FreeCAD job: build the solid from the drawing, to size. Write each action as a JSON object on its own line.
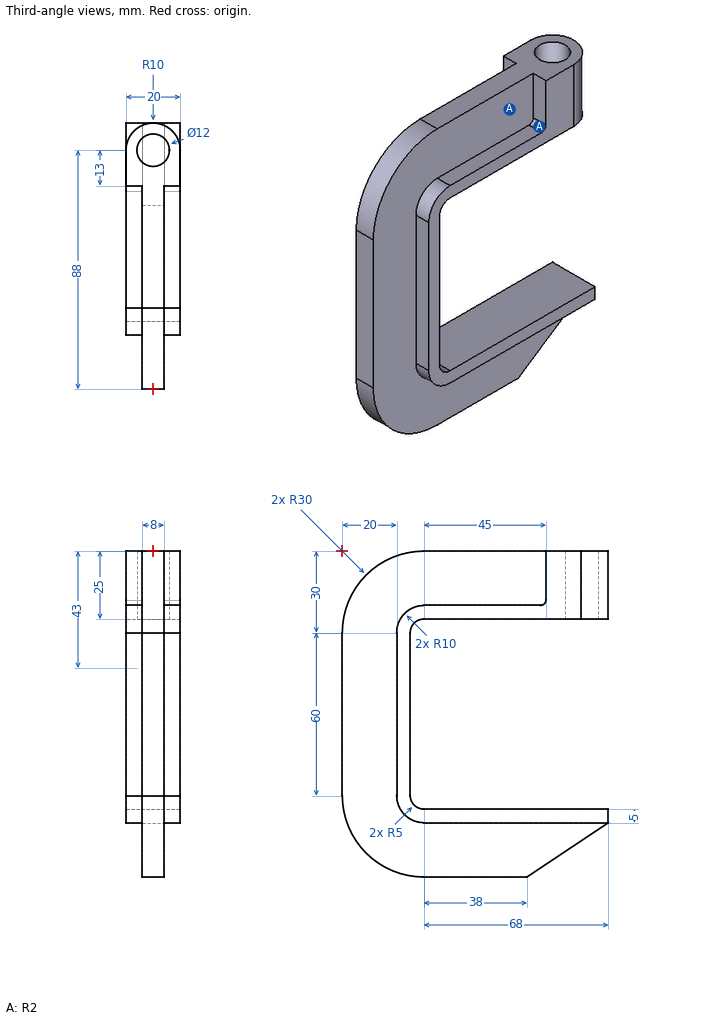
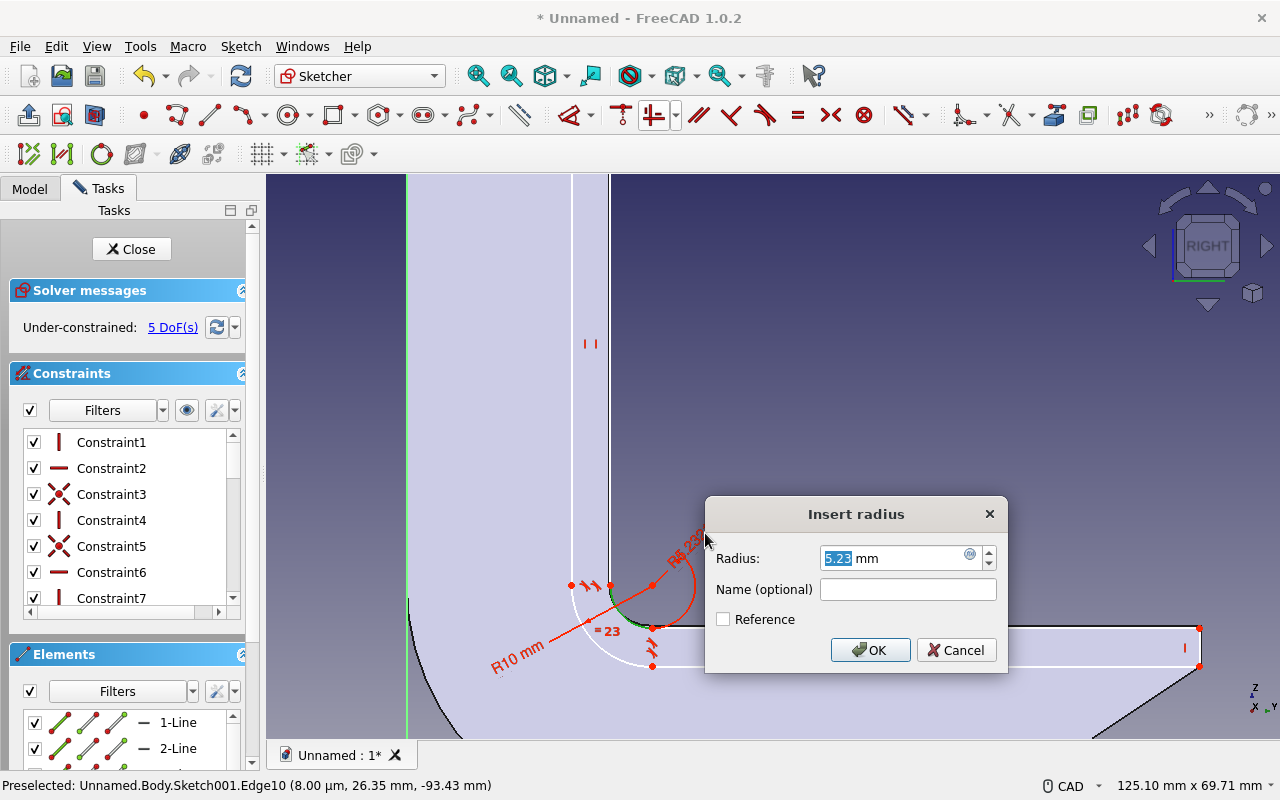
{"action": "type", "text": "5"}
{"action": "key", "text": "Return"}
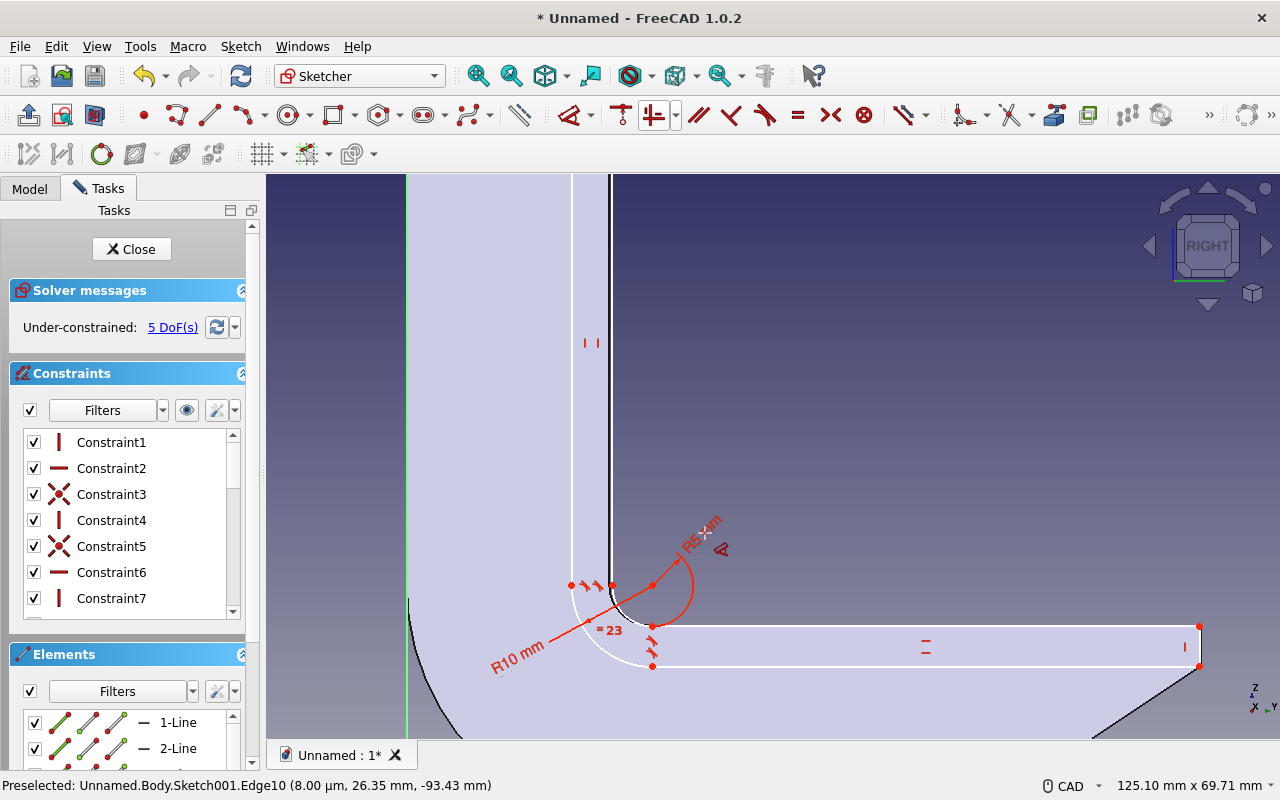
{"action": "left_click", "coordinate": [572, 245]}
{"action": "left_click", "coordinate": [538, 394]}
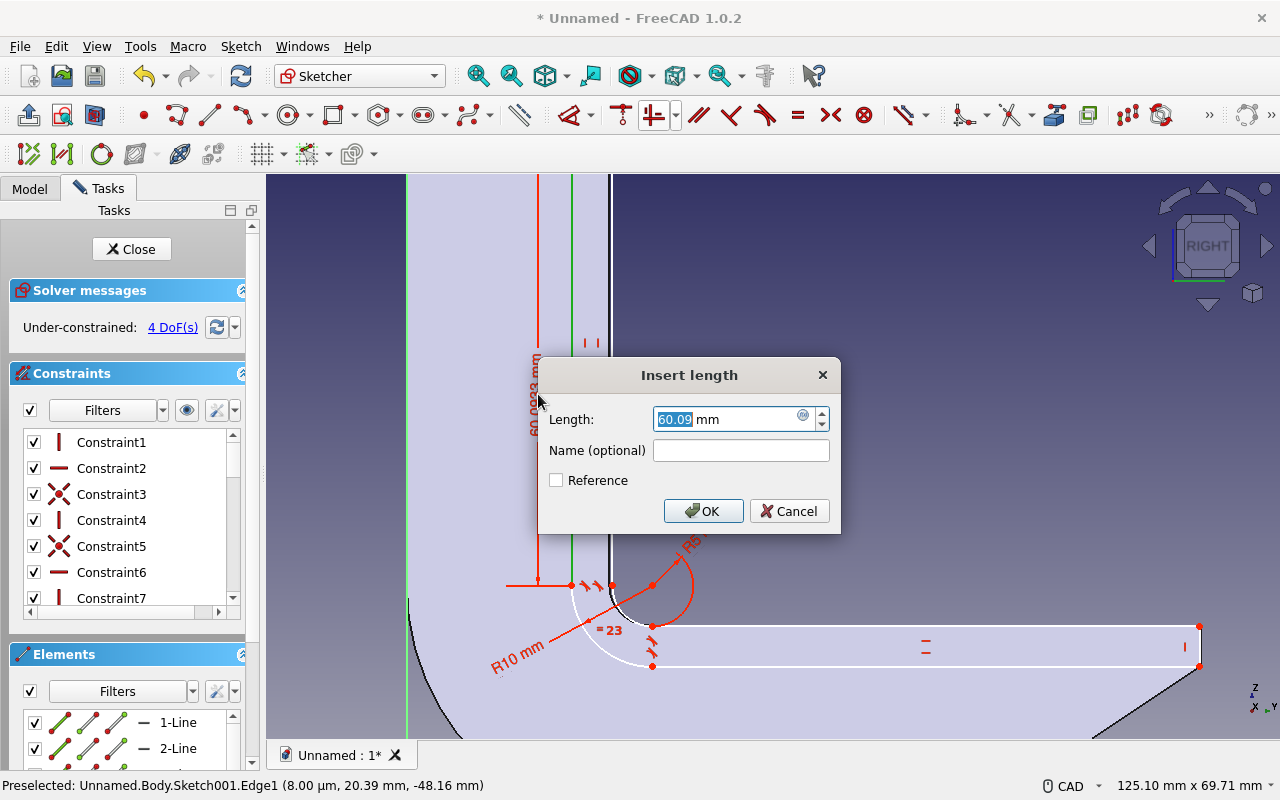
{"action": "type", "text": "60"}
{"action": "key", "text": "Return"}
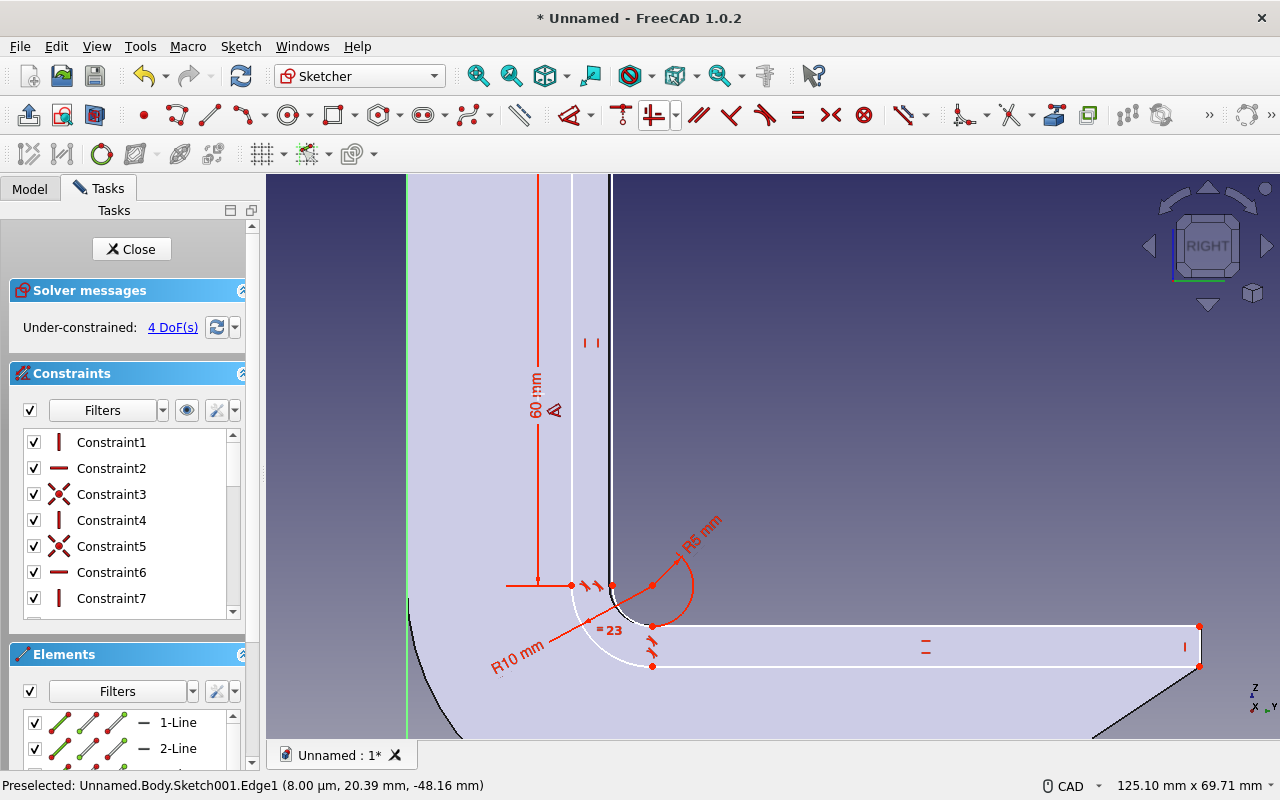
{"action": "left_click", "coordinate": [817, 667]}
{"action": "left_click", "coordinate": [884, 701]}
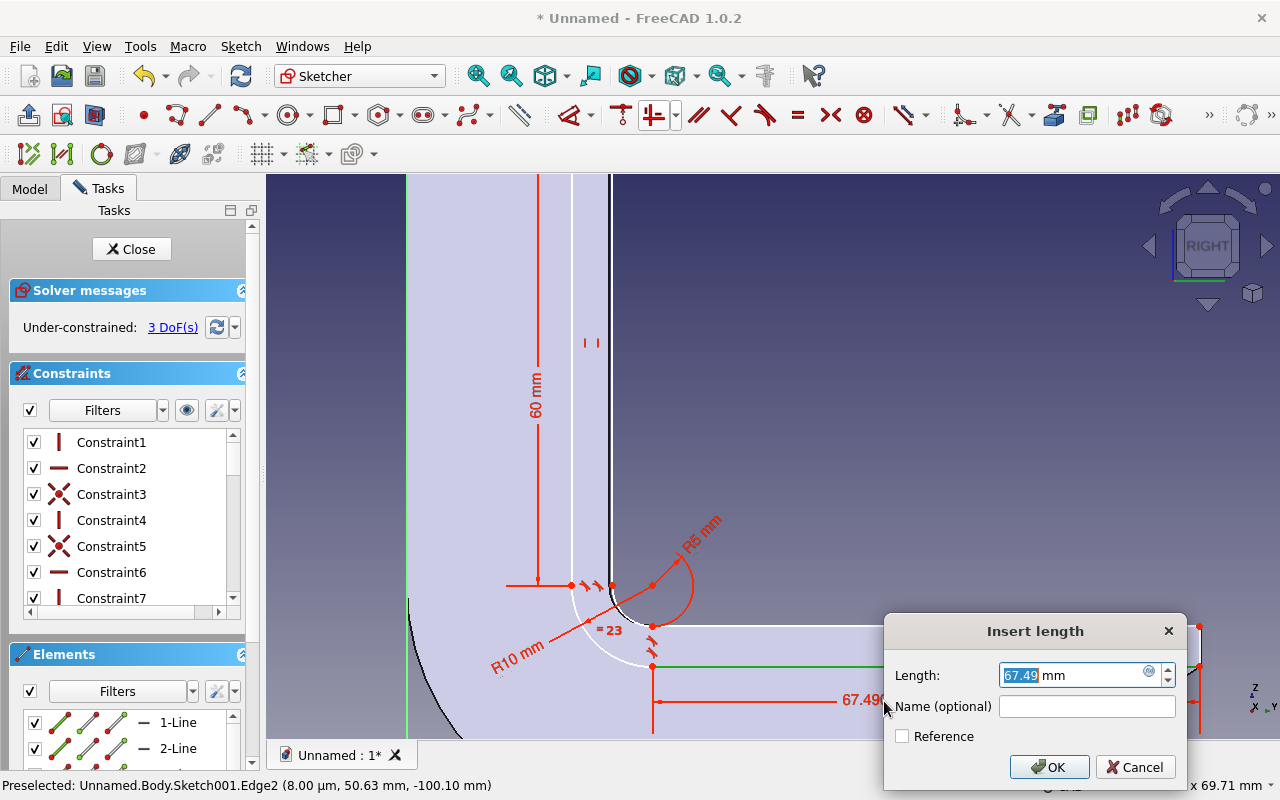
{"action": "type", "text": "68"}
{"action": "key", "text": "Return"}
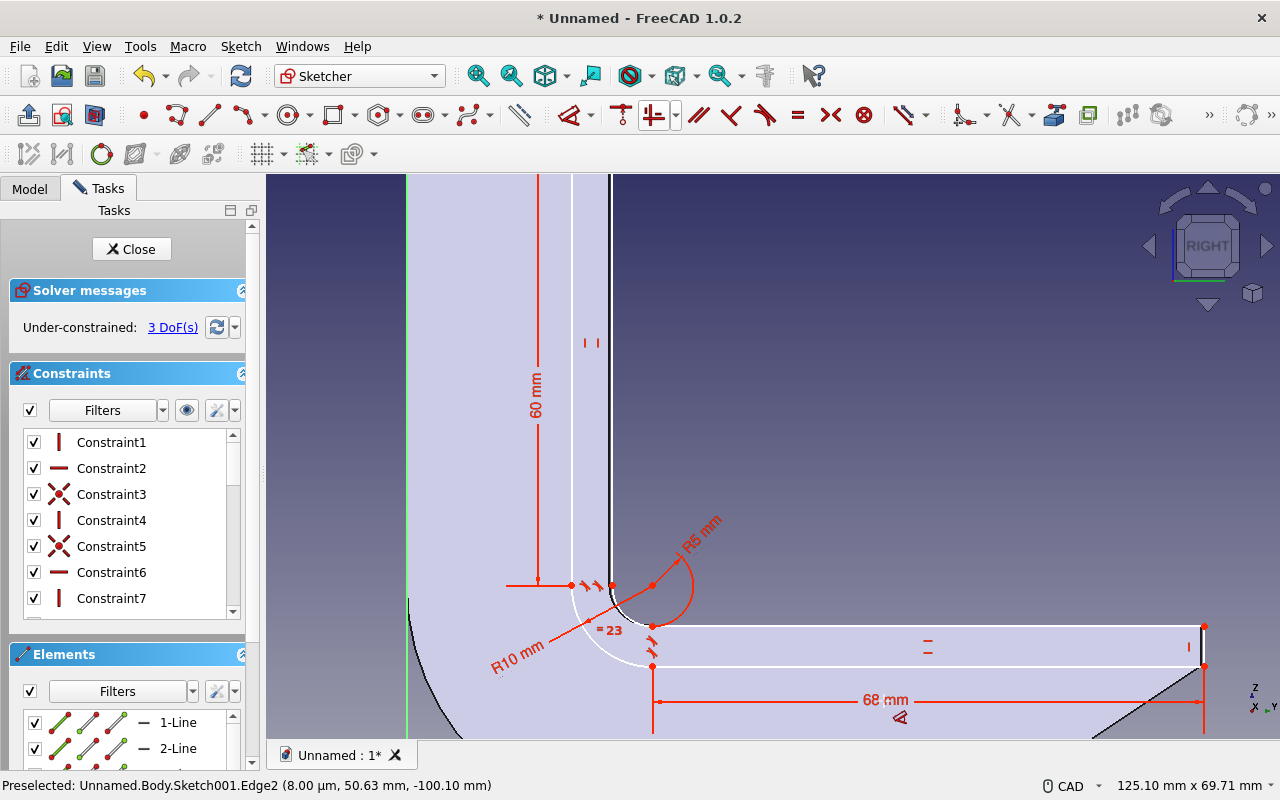
{"action": "scroll", "coordinate": [623, 616], "scroll_direction": "down", "scroll_amount": 4}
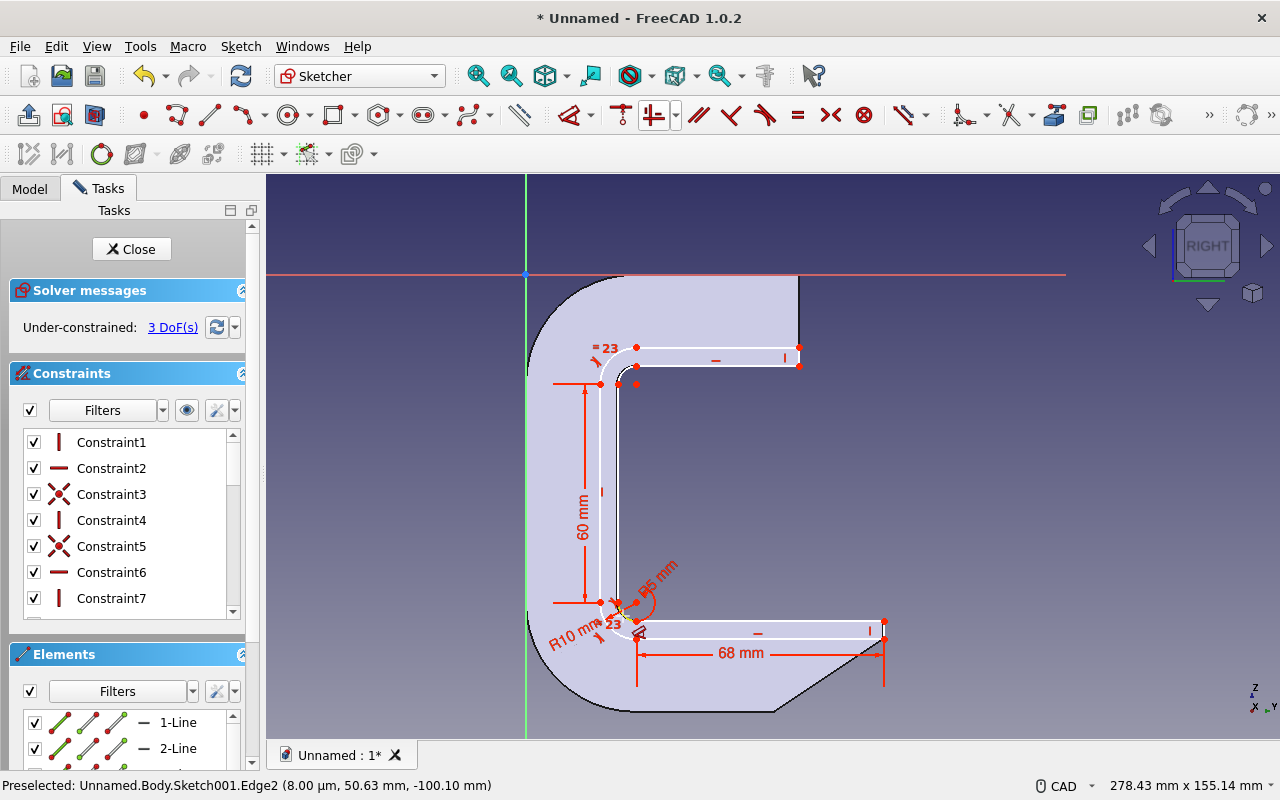
{"action": "left_click", "coordinate": [685, 366]}
{"action": "left_click", "coordinate": [718, 332]}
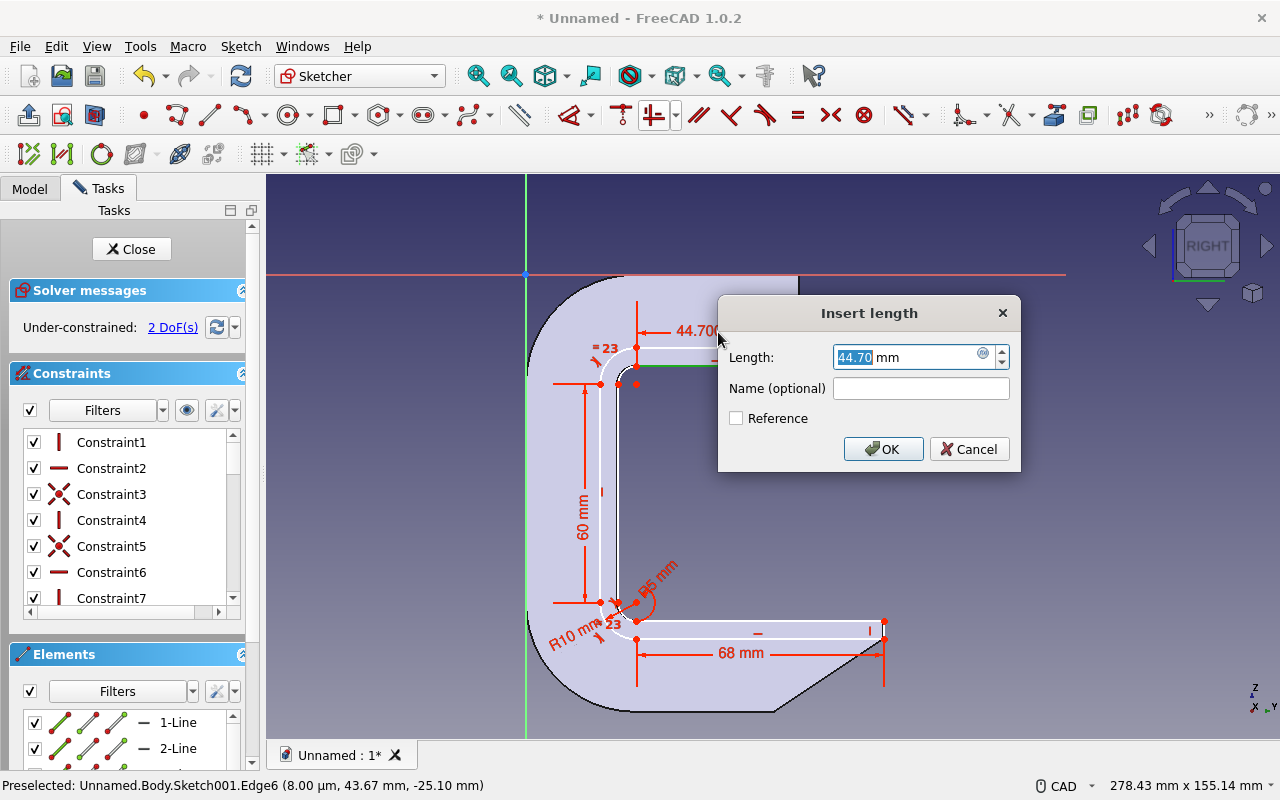
{"action": "type", "text": "45"}
{"action": "key", "text": "Return"}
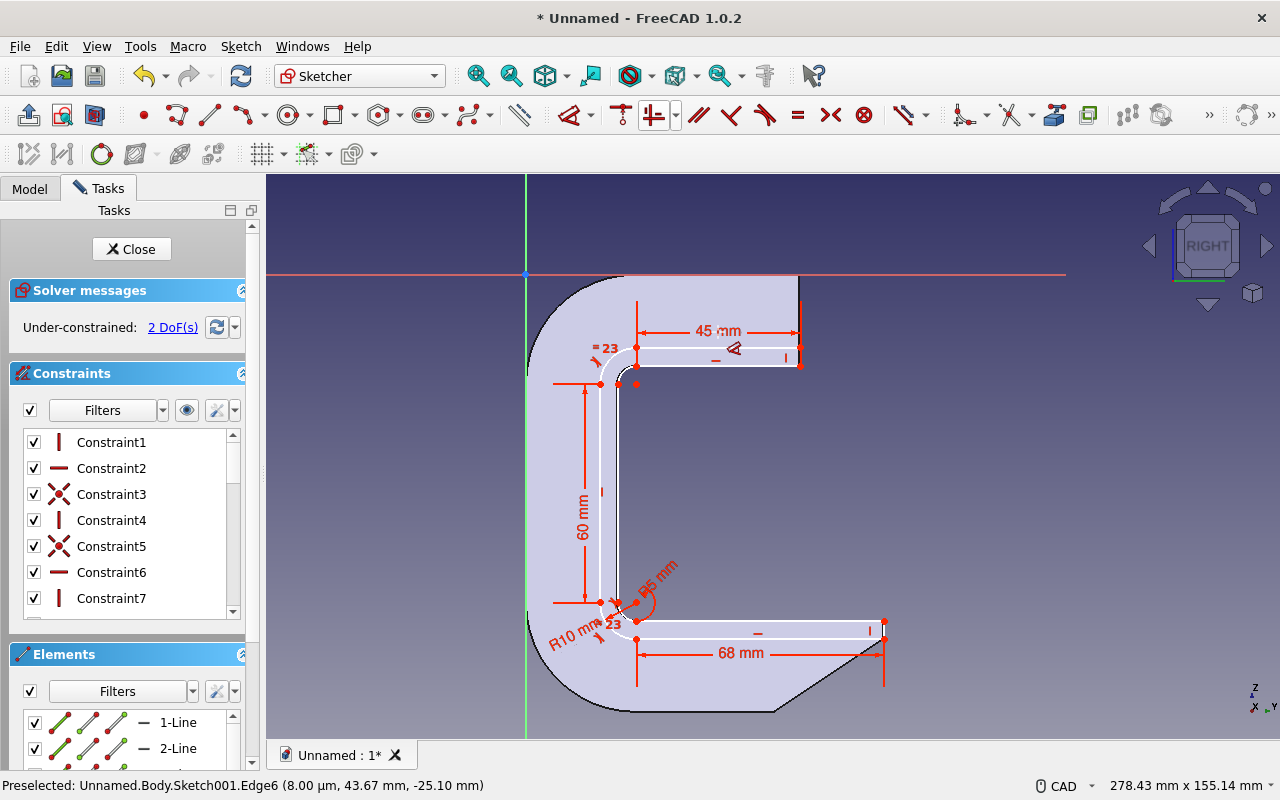
{"action": "left_click", "coordinate": [600, 384]}
{"action": "left_click", "coordinate": [563, 241]}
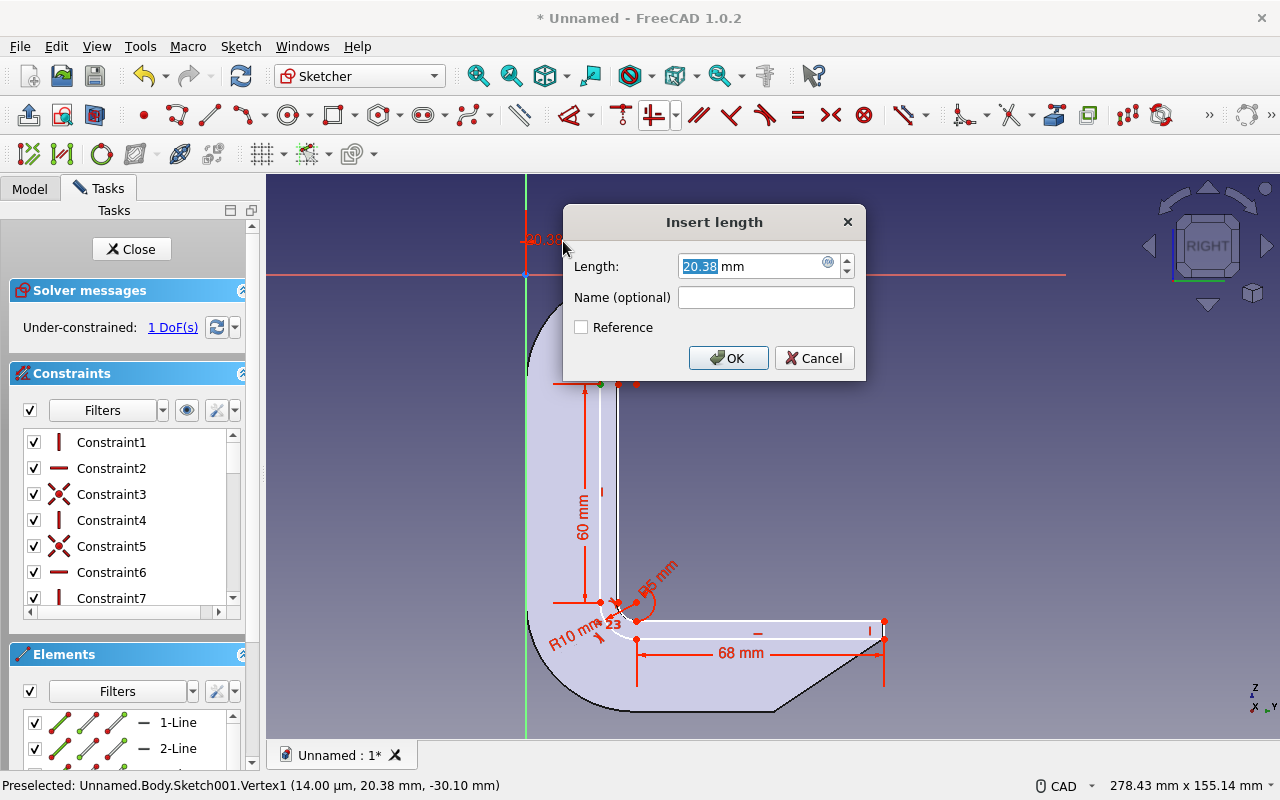
{"action": "type", "text": "20"}
{"action": "key", "text": "Return"}